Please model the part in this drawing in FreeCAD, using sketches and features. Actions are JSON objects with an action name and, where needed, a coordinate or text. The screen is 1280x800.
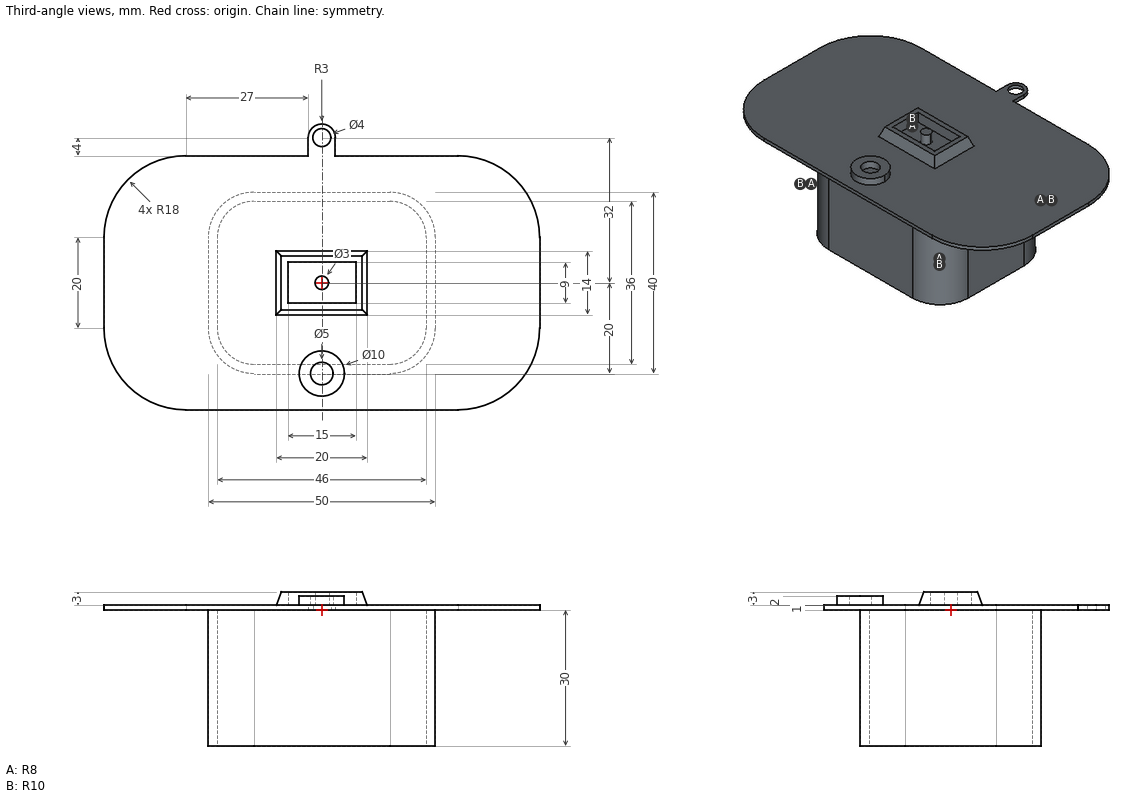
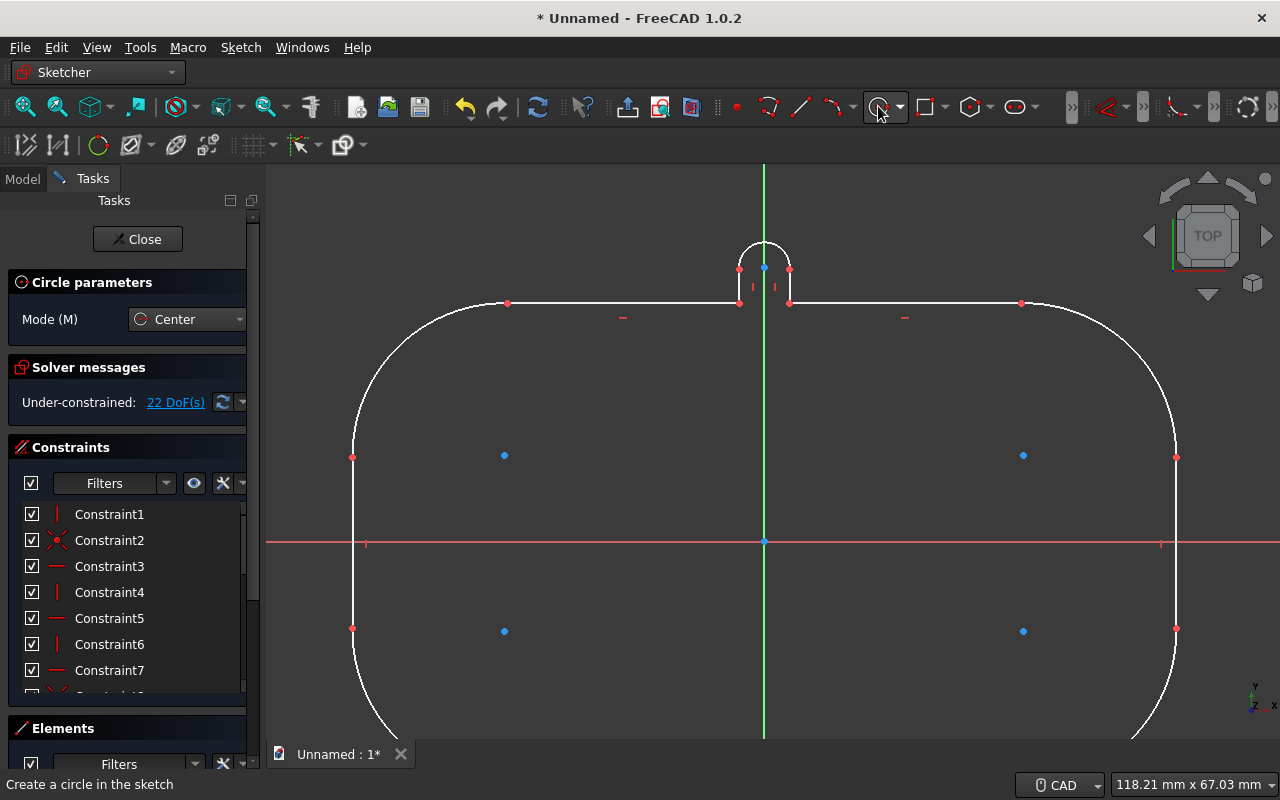
{"action": "scroll", "coordinate": [764, 267], "scroll_direction": "up", "scroll_amount": 2}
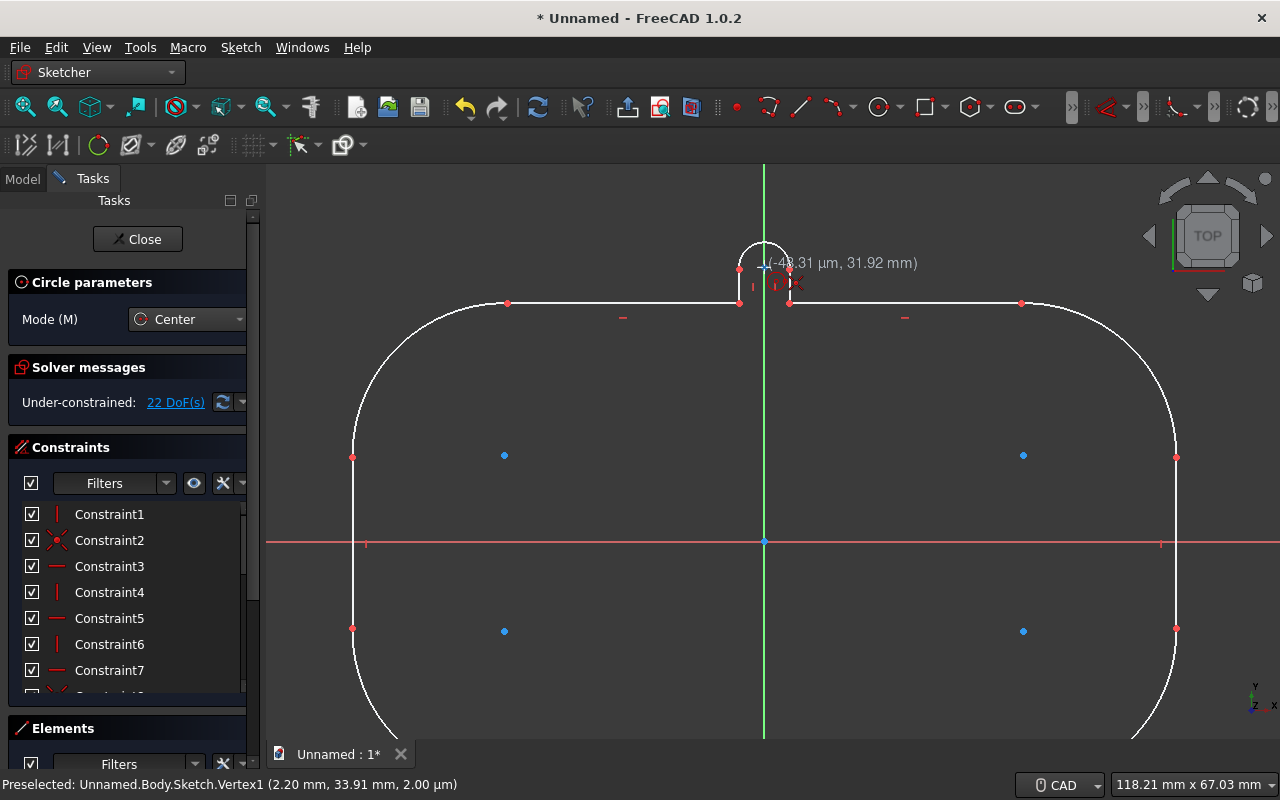
{"action": "left_click", "coordinate": [764, 267]}
{"action": "mouse_move", "coordinate": [782, 286]}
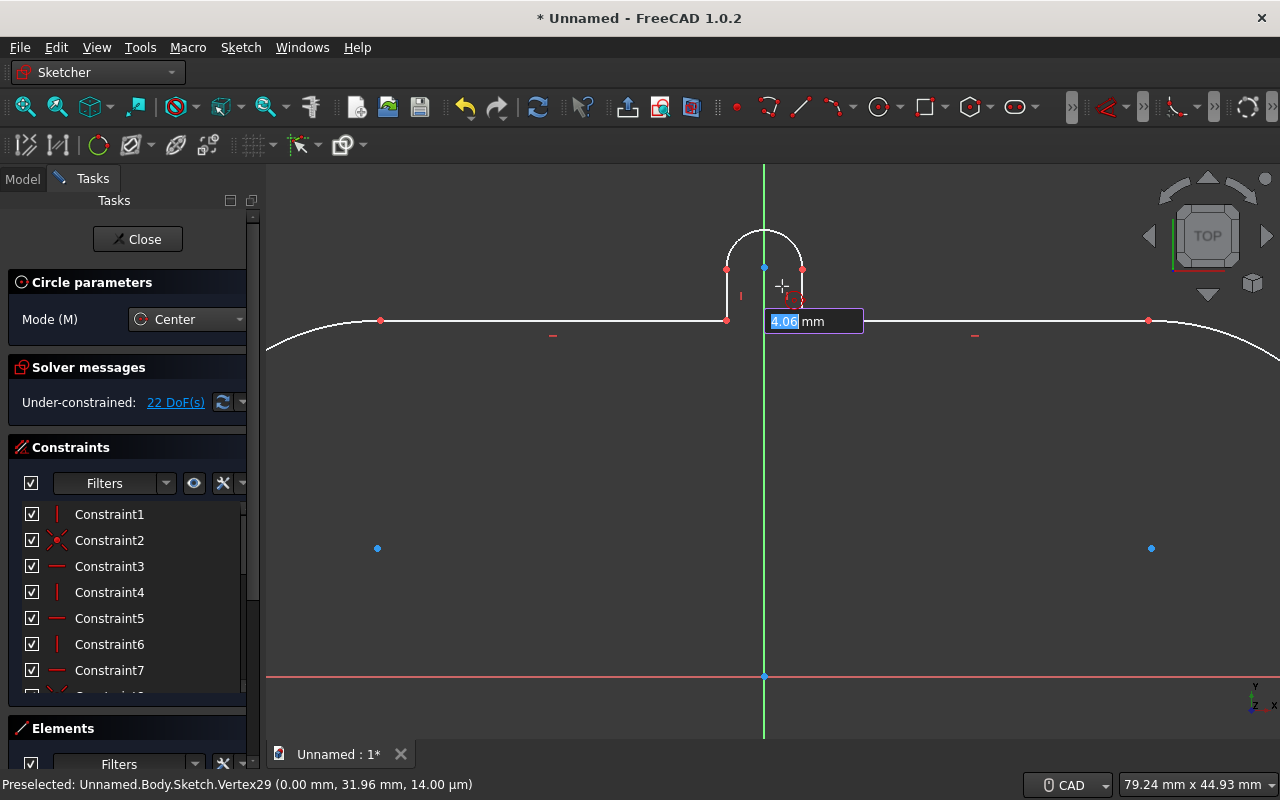
{"action": "type", "text": "4"}
{"action": "key", "text": "Return"}
{"action": "key", "text": "Escape"}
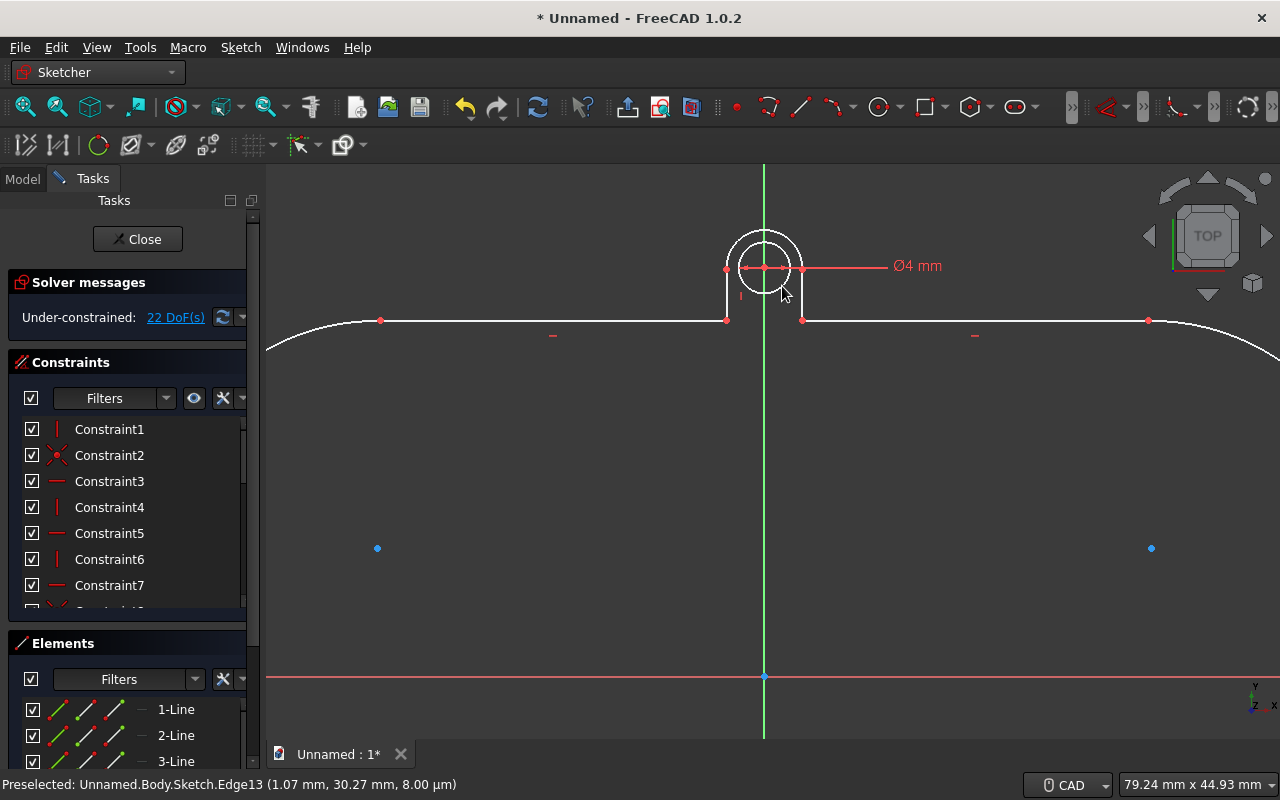
{"action": "left_click", "coordinate": [727, 285]}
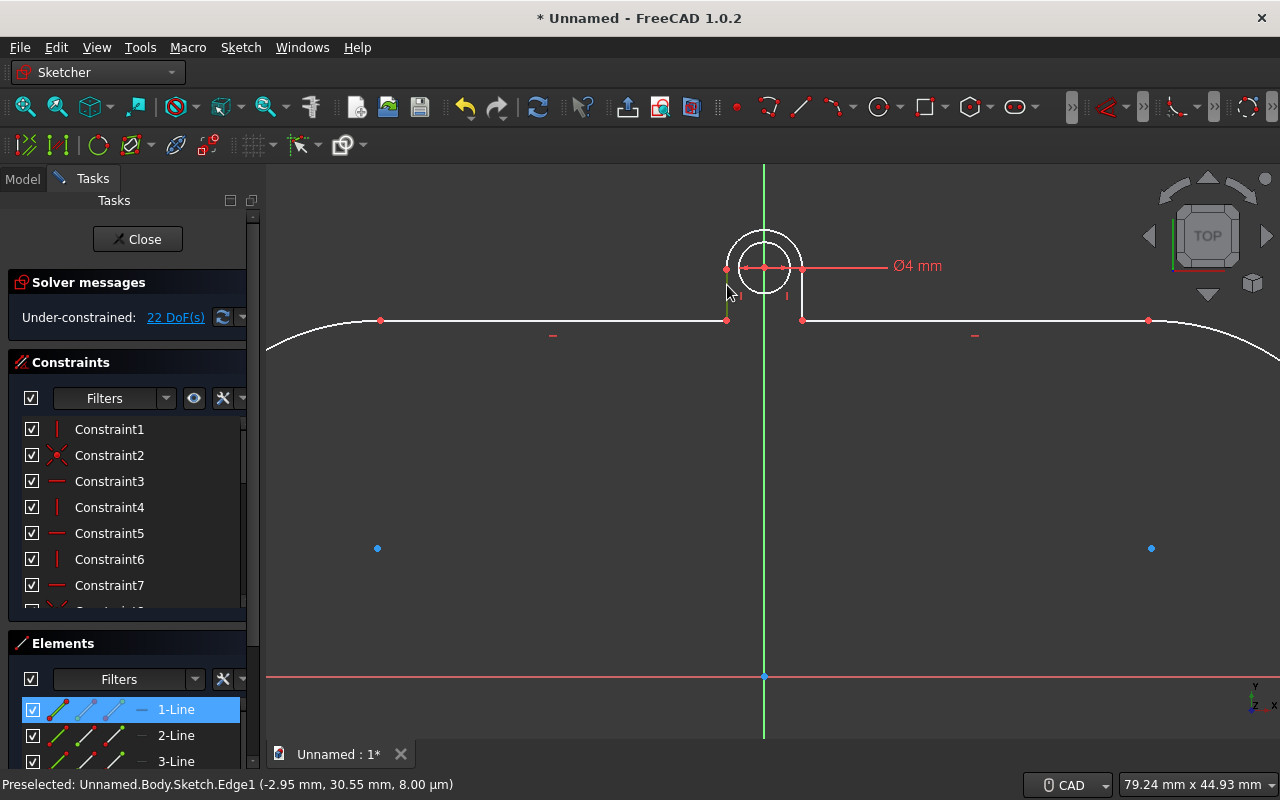
{"action": "left_click", "coordinate": [787, 238]}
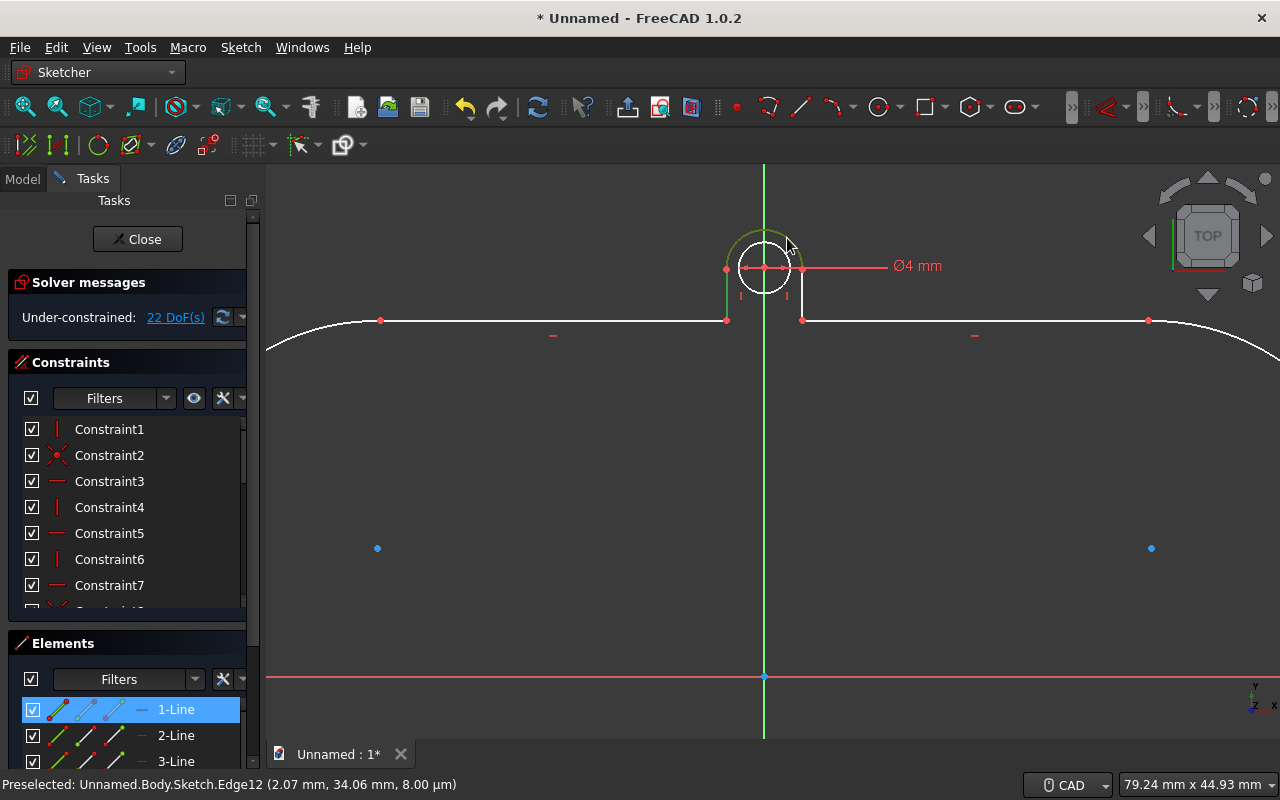
{"action": "key", "text": "t"}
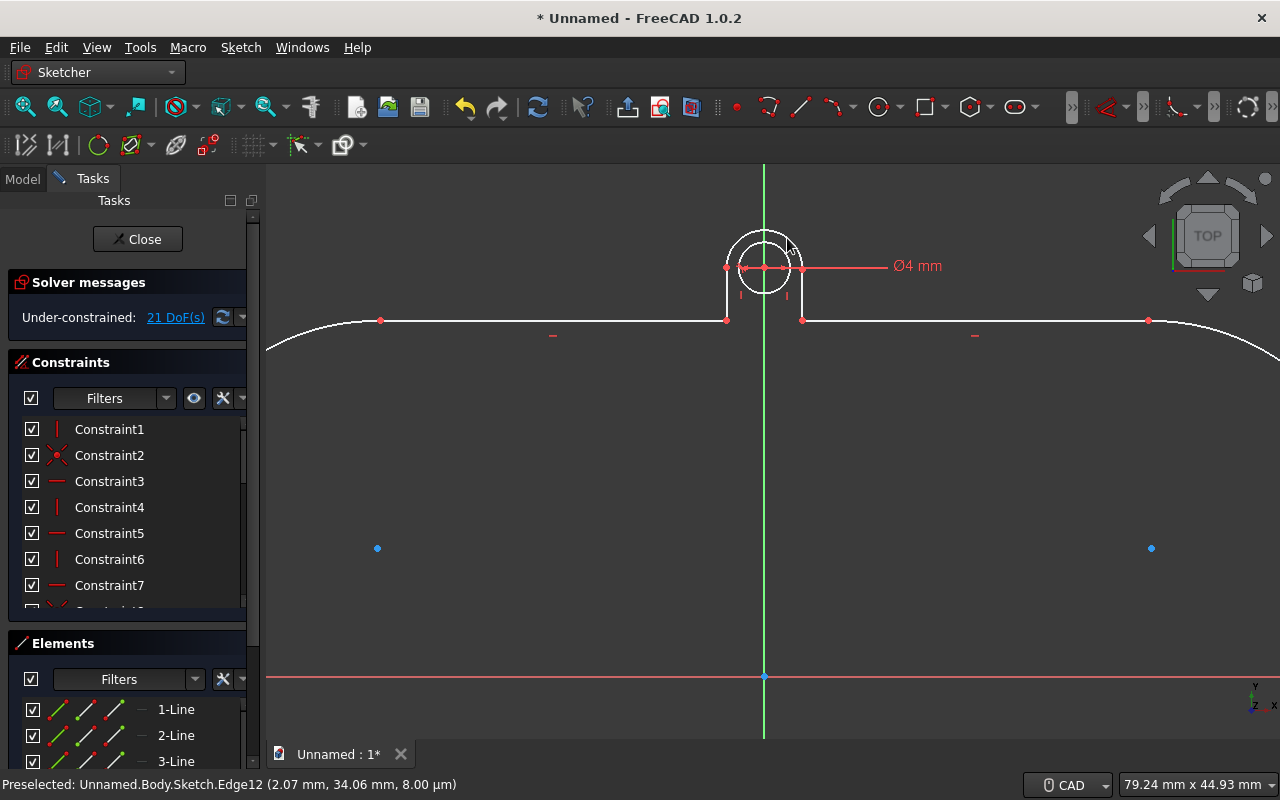
{"action": "left_click", "coordinate": [623, 321]}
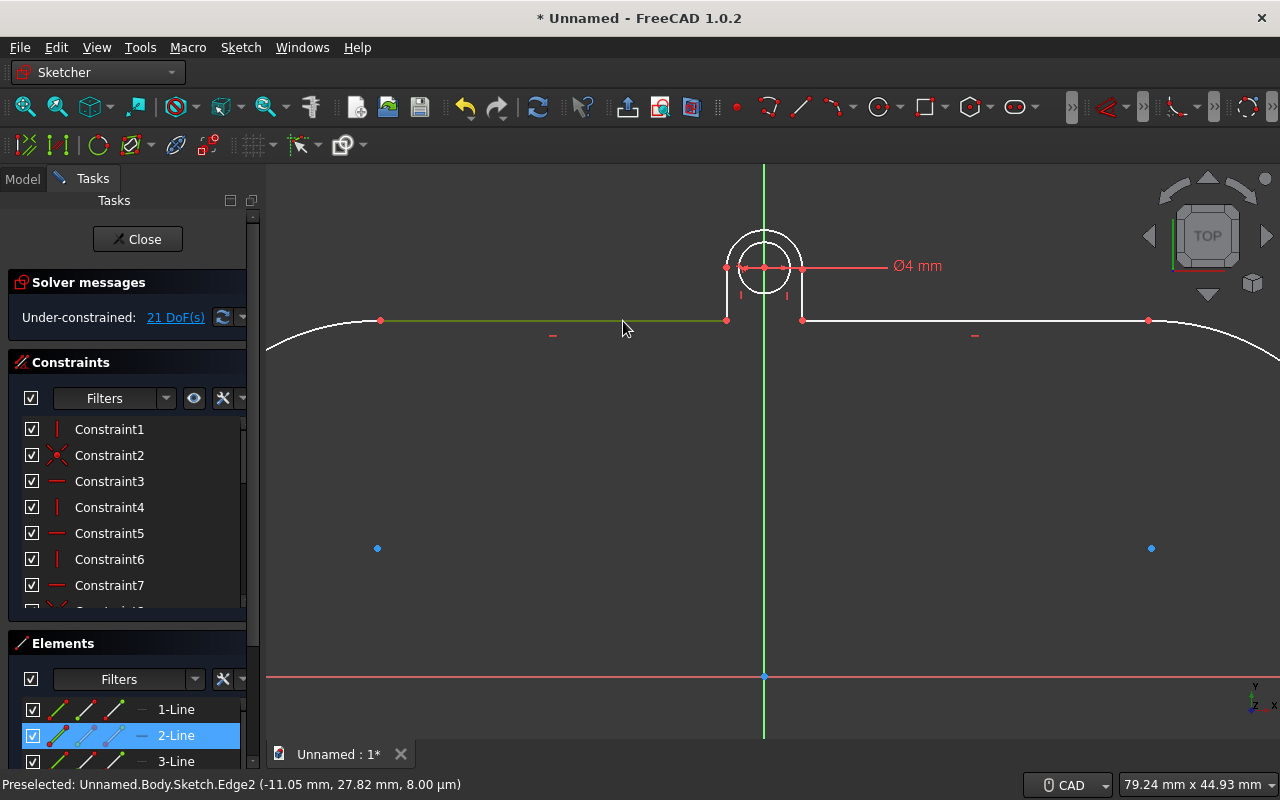
{"action": "left_click", "coordinate": [309, 331]}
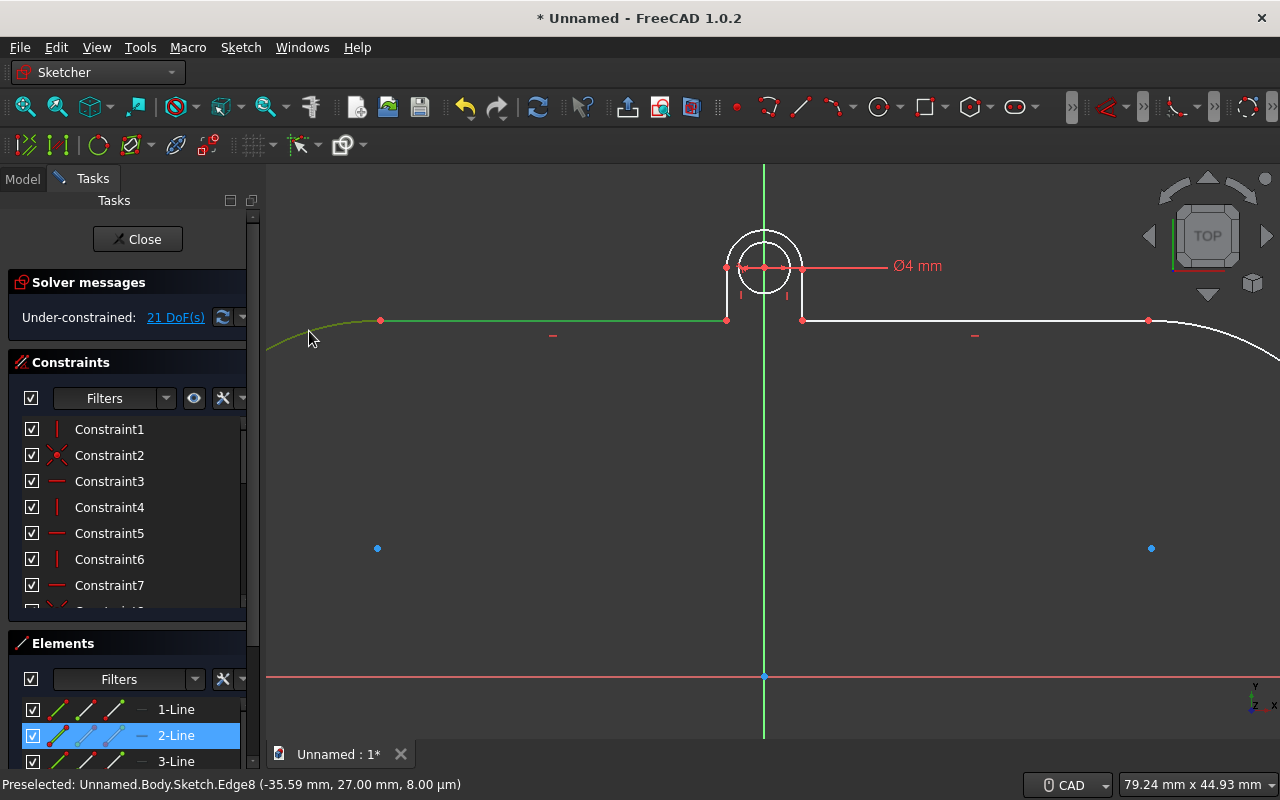
{"action": "key", "text": "t"}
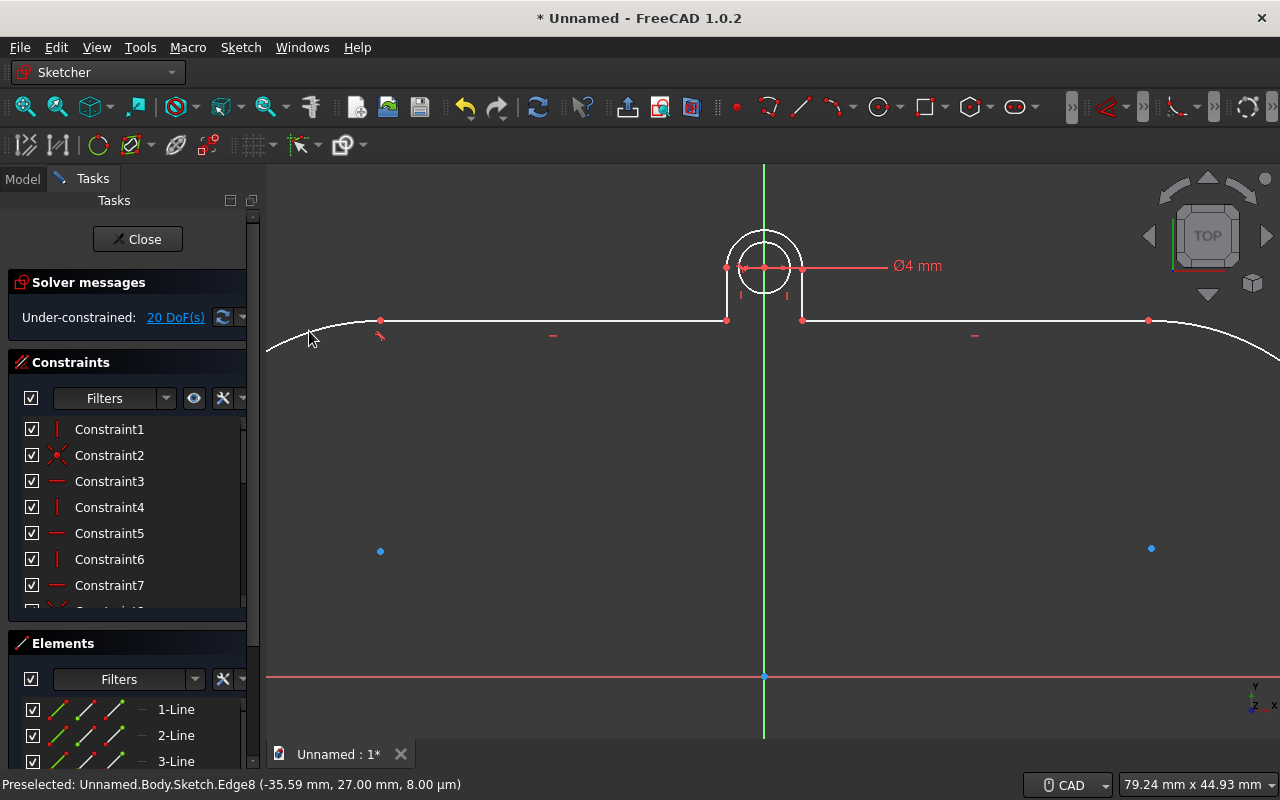
{"action": "scroll", "coordinate": [656, 304], "scroll_direction": "down", "scroll_amount": 4}